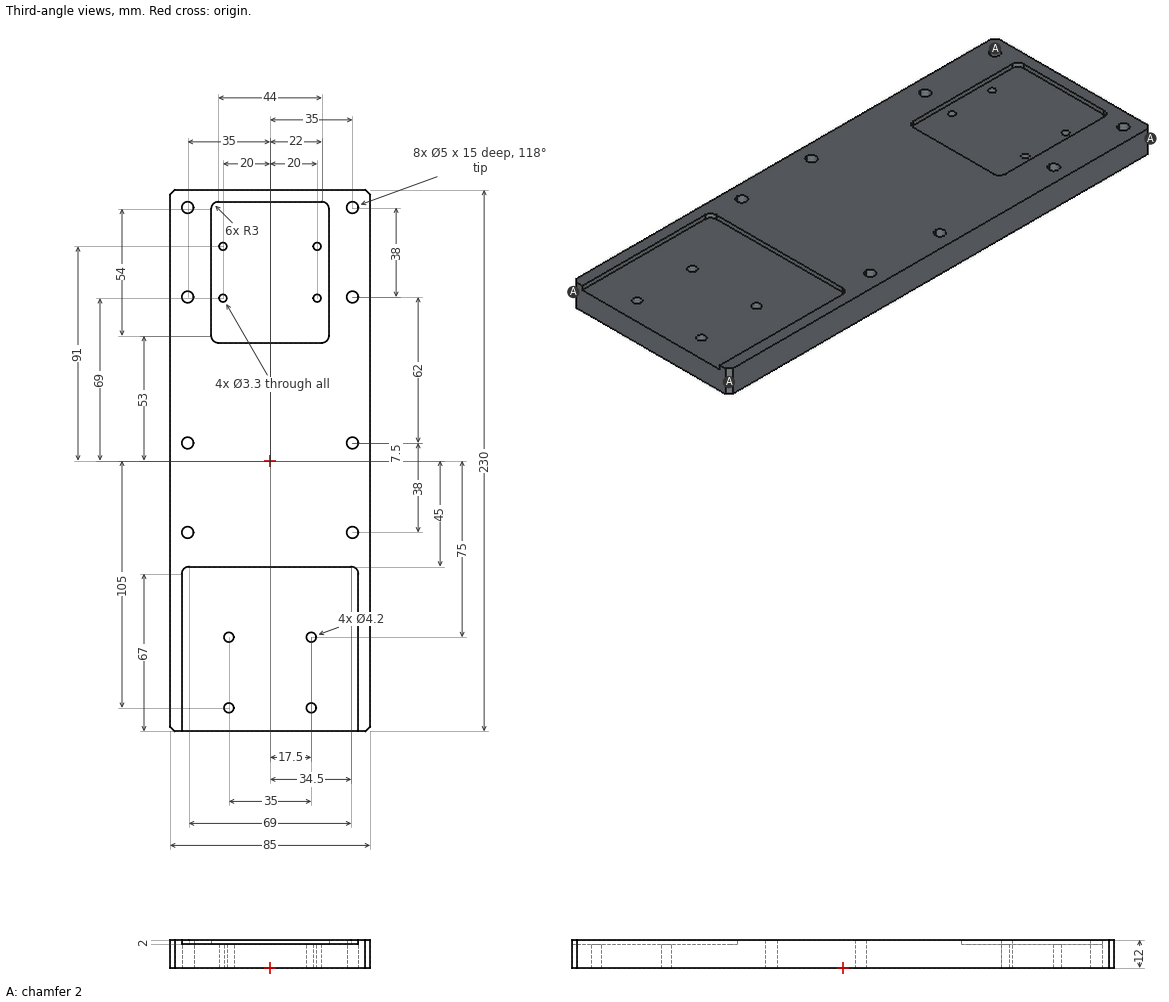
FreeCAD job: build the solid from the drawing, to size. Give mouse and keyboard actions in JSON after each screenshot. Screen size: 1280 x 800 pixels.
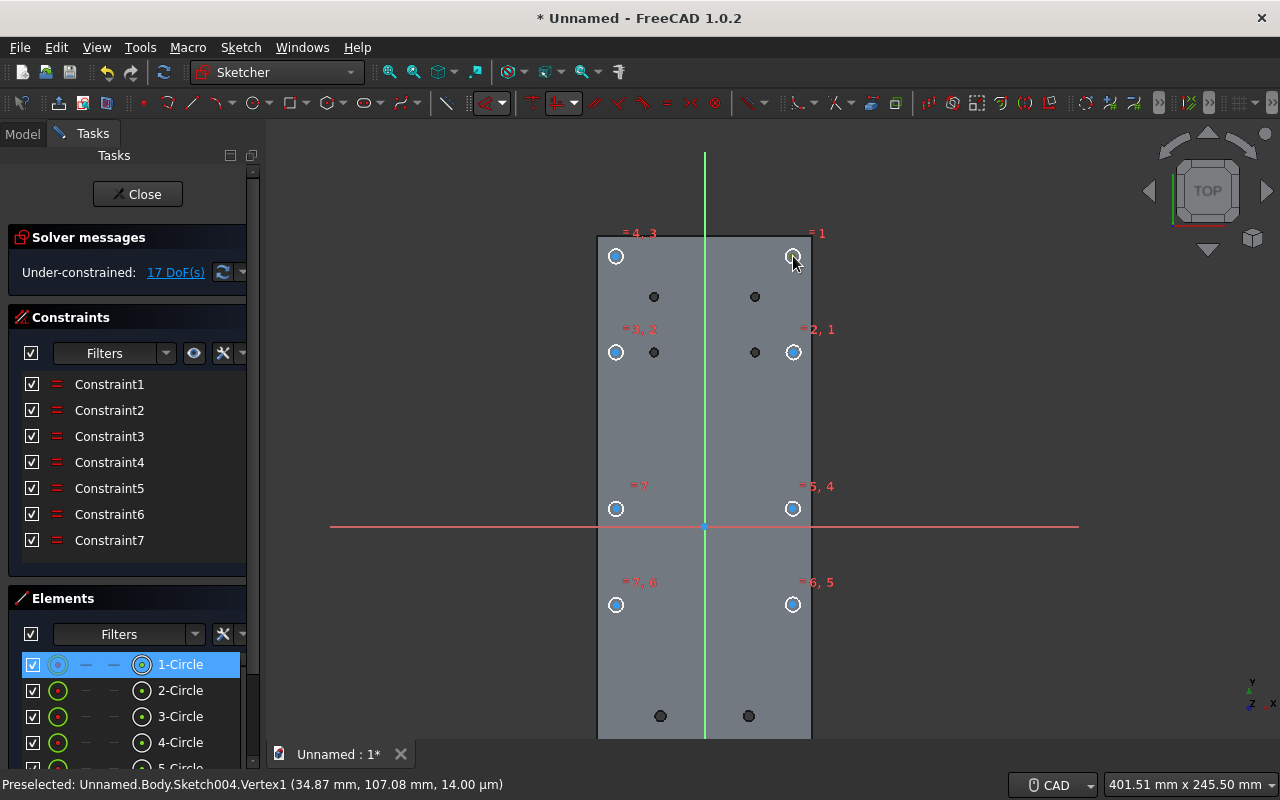
{"action": "left_click", "coordinate": [794, 352]}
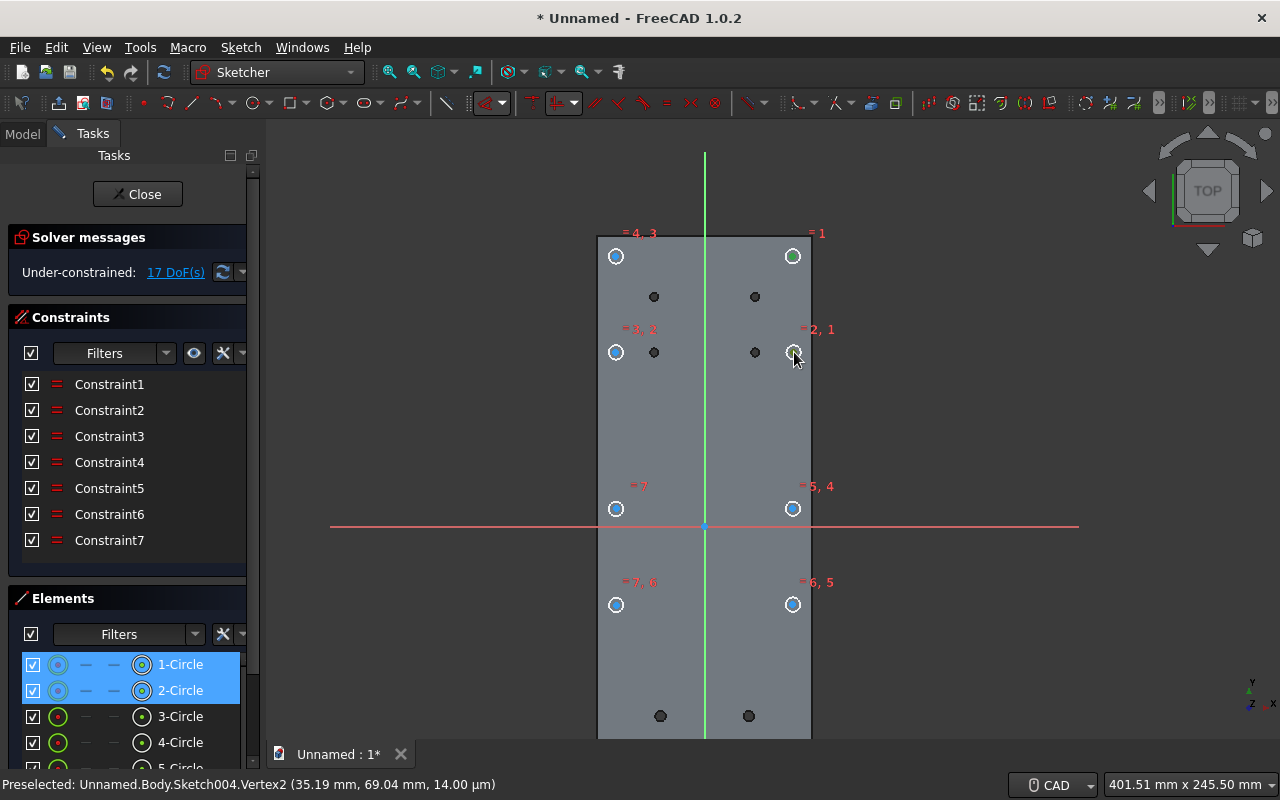
{"action": "left_click", "coordinate": [576, 104]}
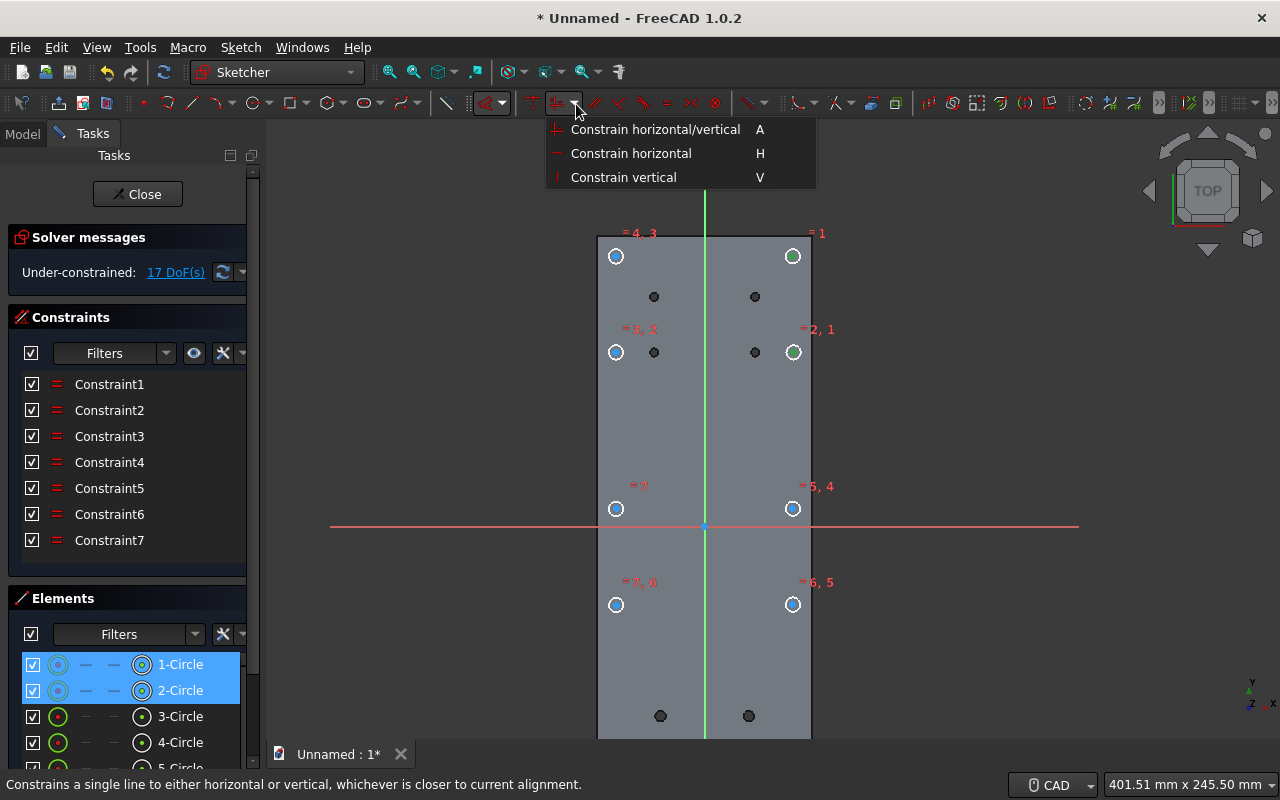
{"action": "left_click", "coordinate": [681, 177]}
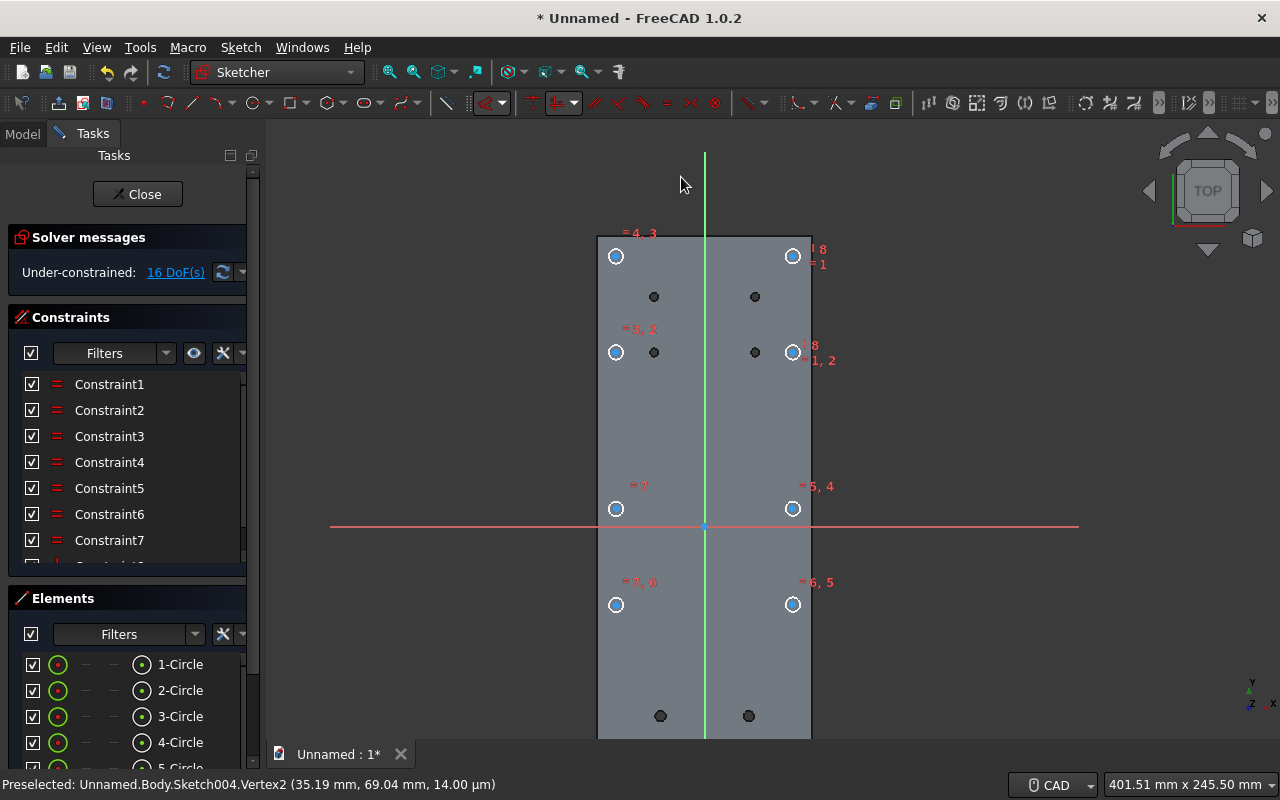
{"action": "left_click", "coordinate": [793, 352]}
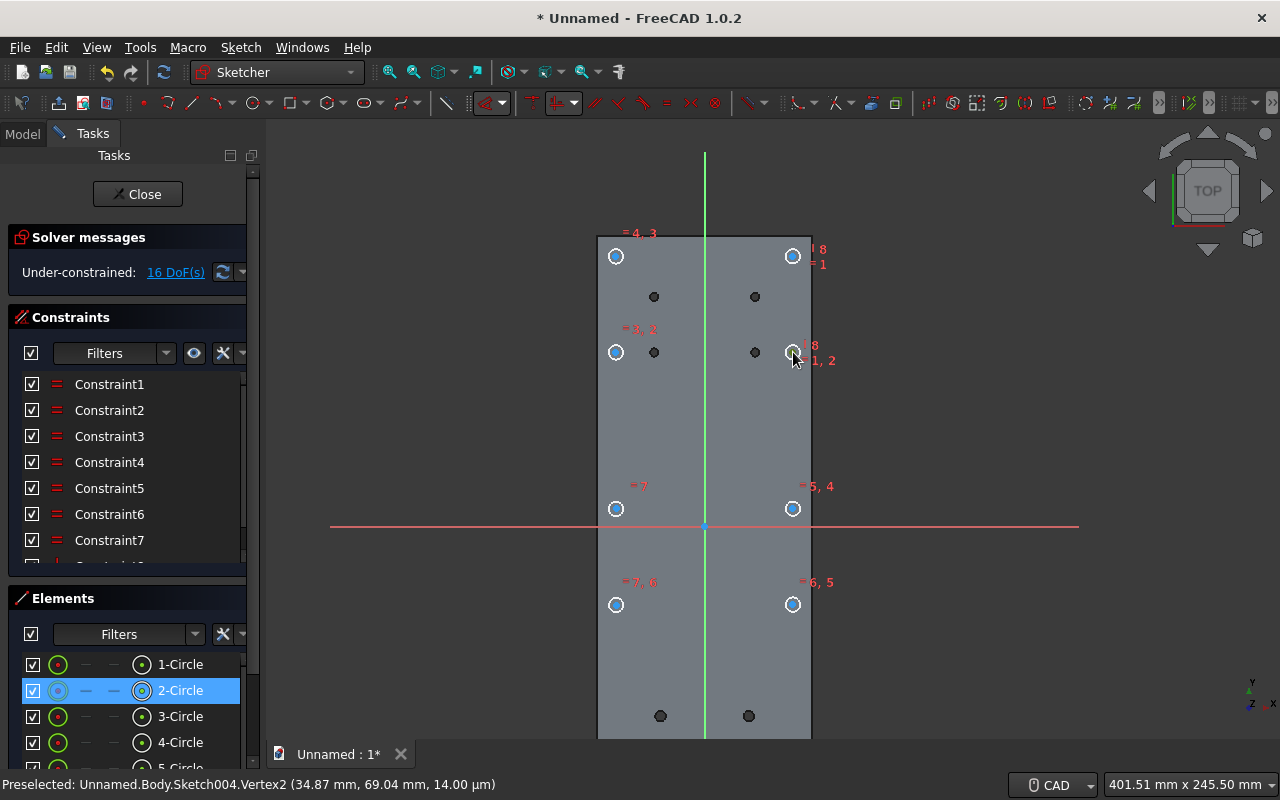
{"action": "left_click", "coordinate": [616, 352]}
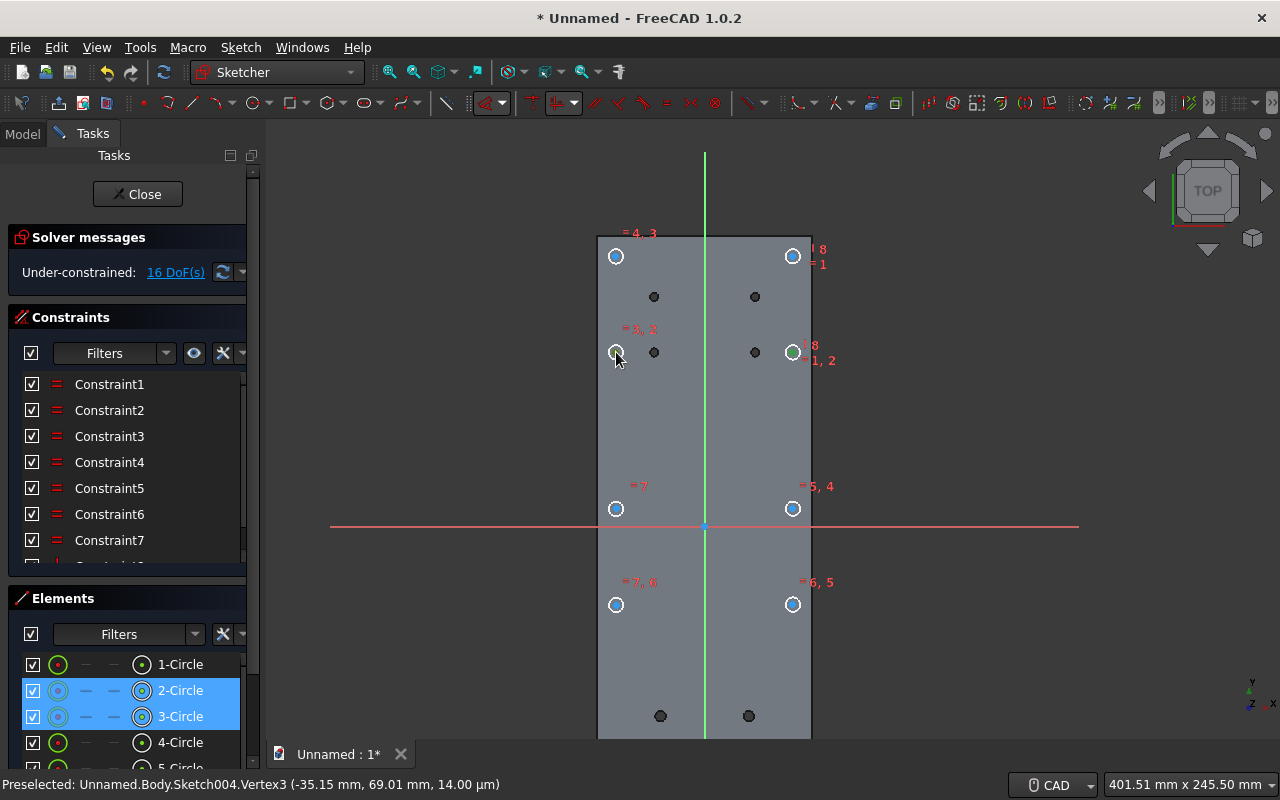
{"action": "left_click", "coordinate": [576, 104]}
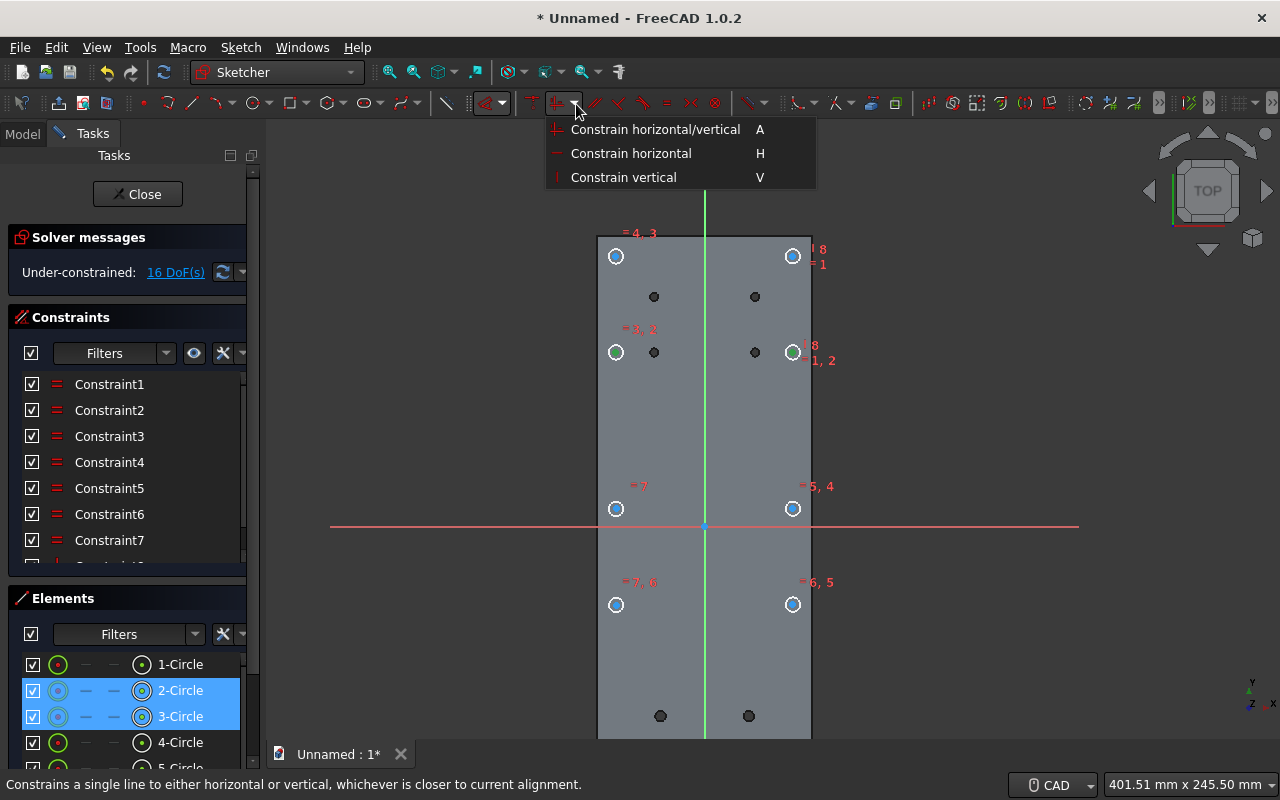
{"action": "left_click", "coordinate": [681, 153]}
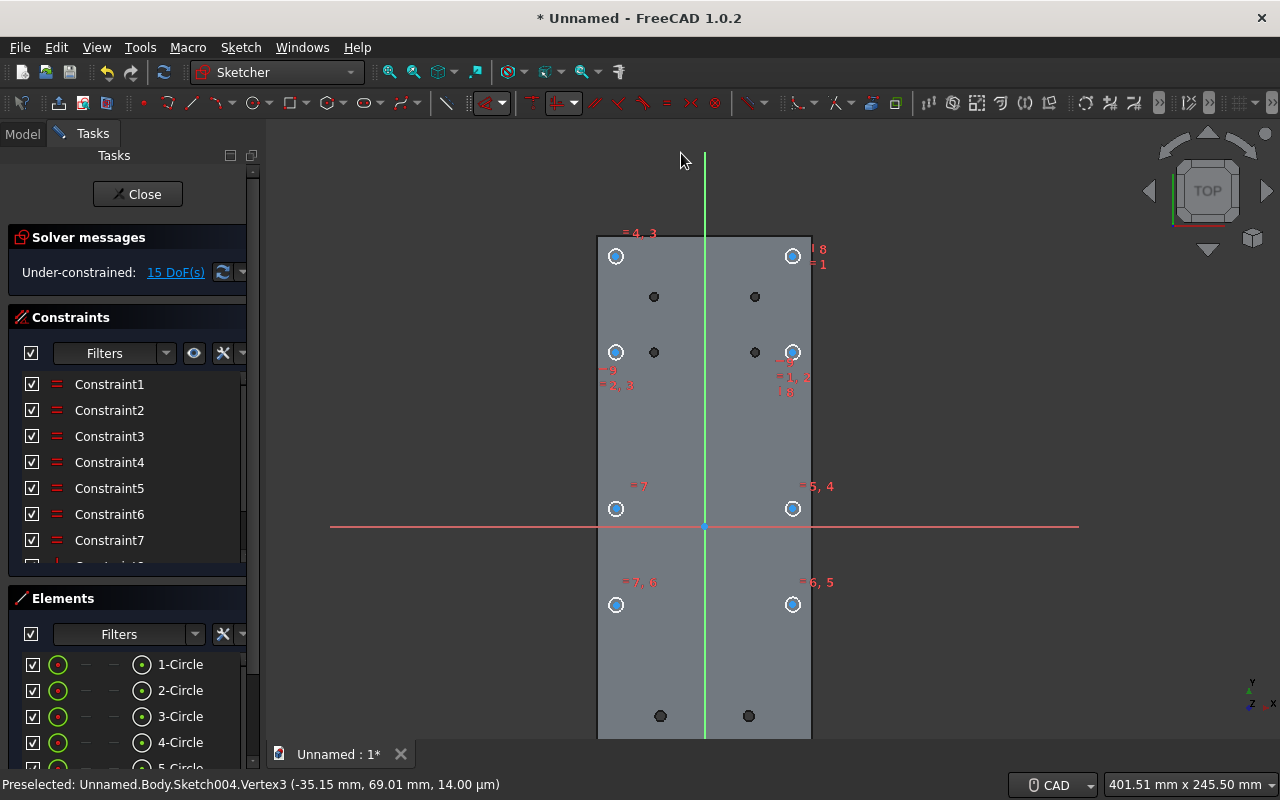
{"action": "left_click", "coordinate": [616, 352]}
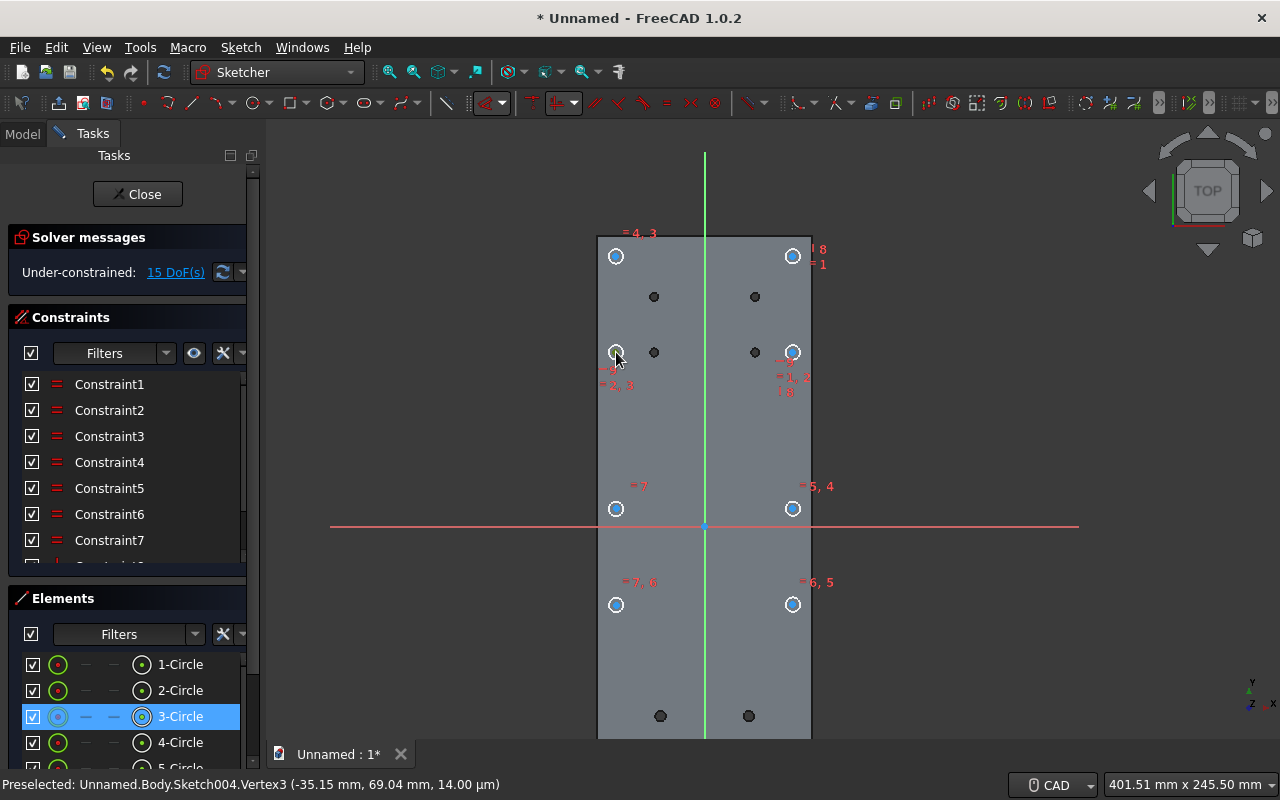
{"action": "left_click", "coordinate": [616, 256]}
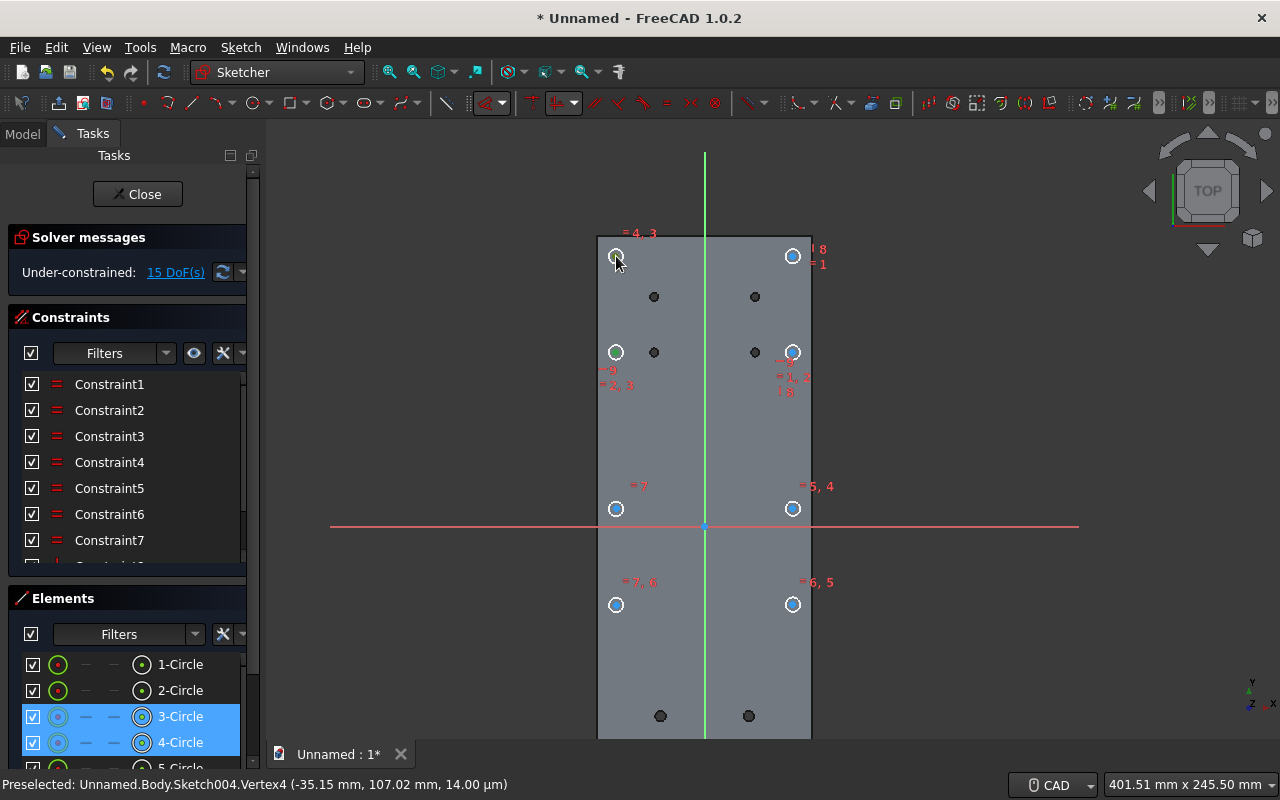
{"action": "left_click", "coordinate": [576, 104]}